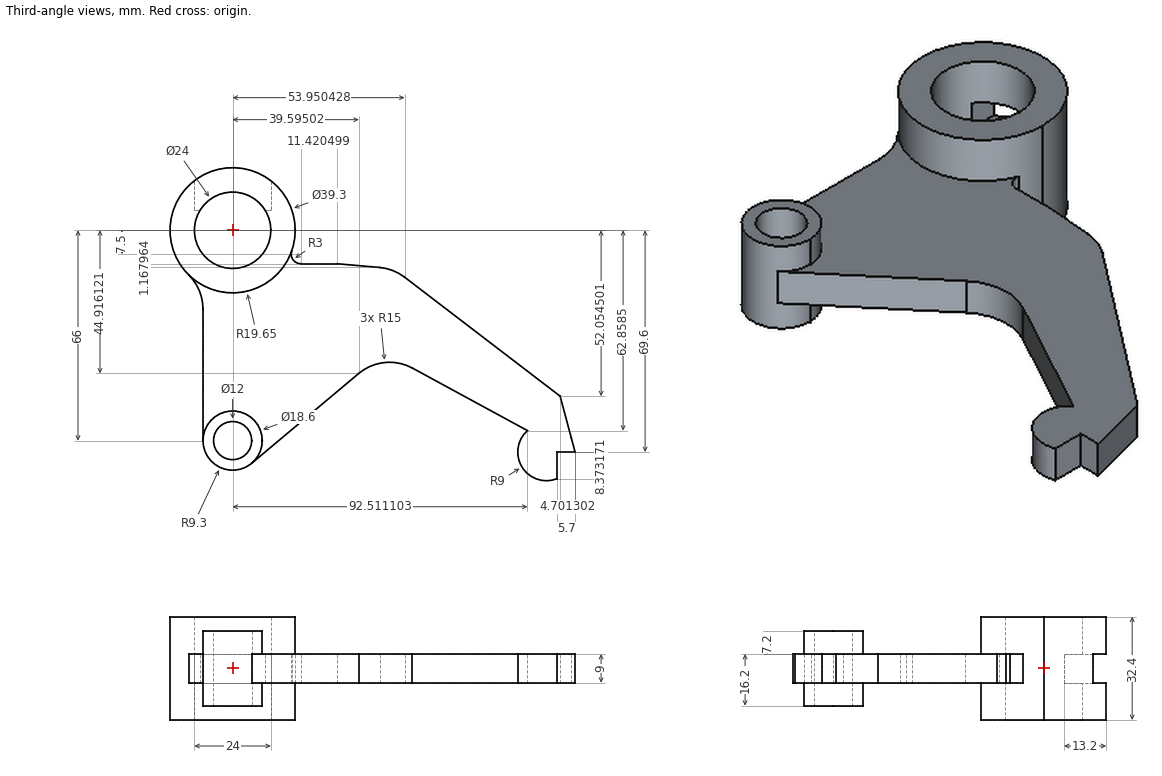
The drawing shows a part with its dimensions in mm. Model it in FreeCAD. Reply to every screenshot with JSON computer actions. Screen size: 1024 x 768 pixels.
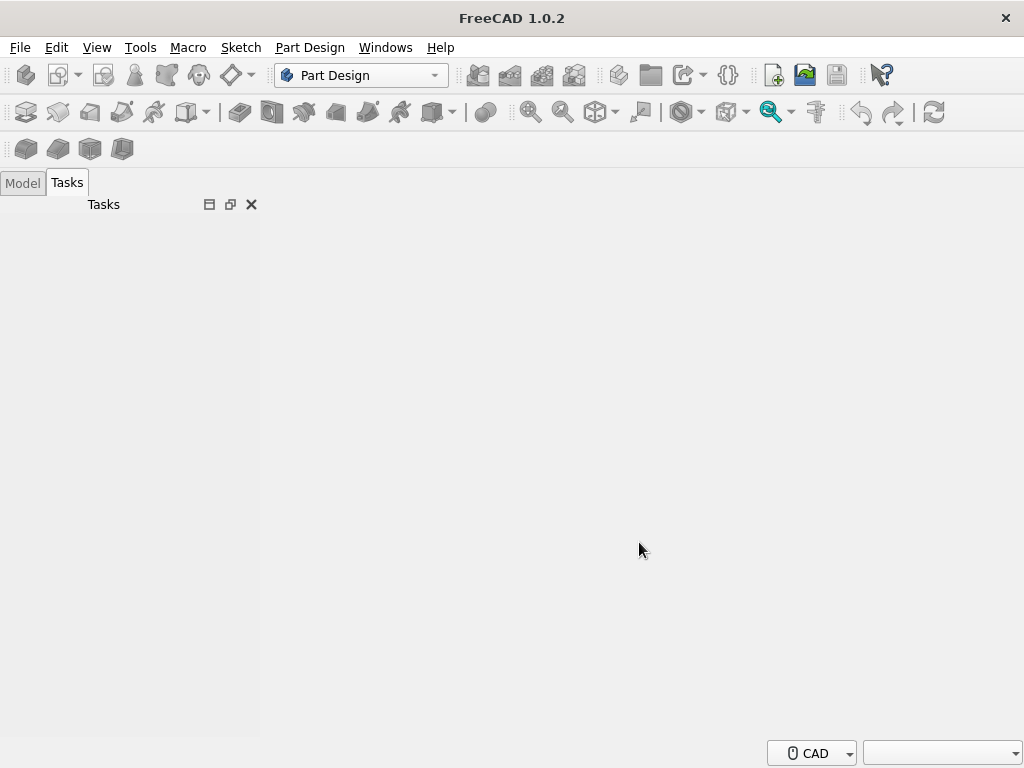
{"action": "key", "text": "ctrl+n"}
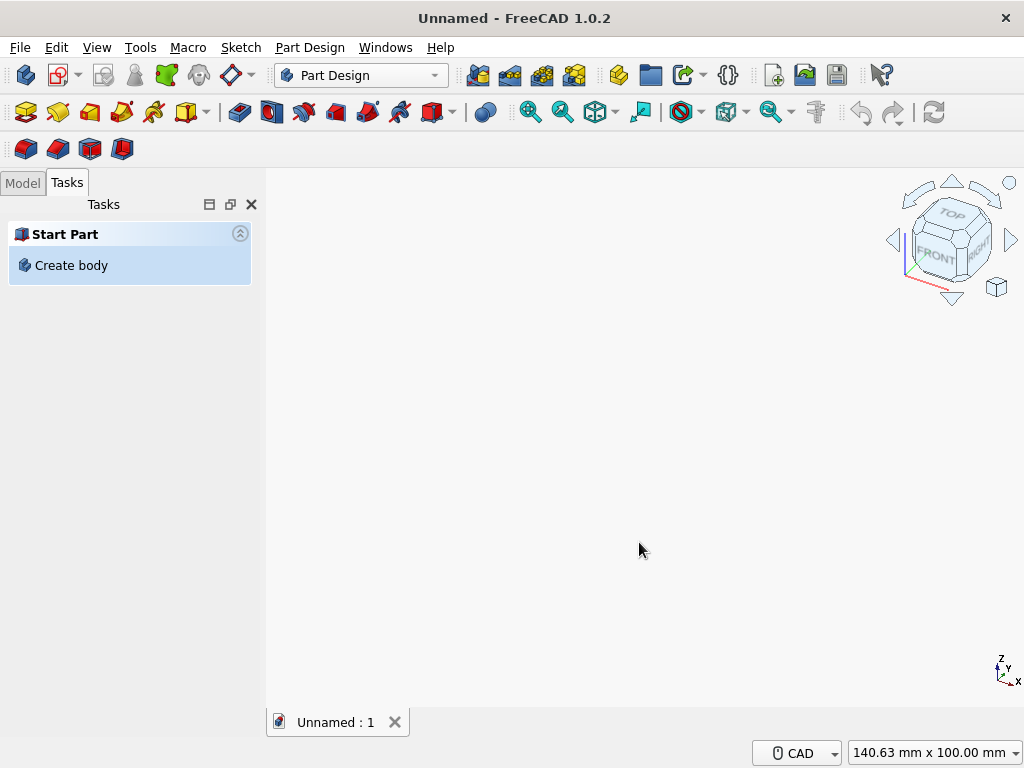
{"action": "left_click", "coordinate": [58, 76]}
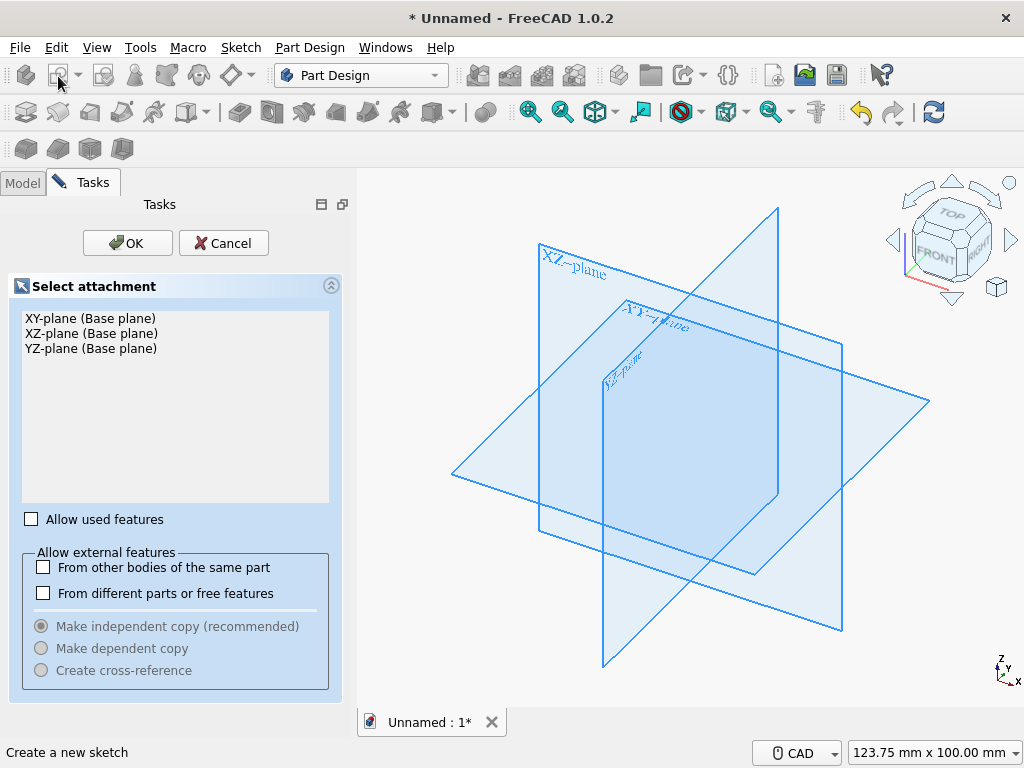
{"action": "left_click", "coordinate": [82, 318]}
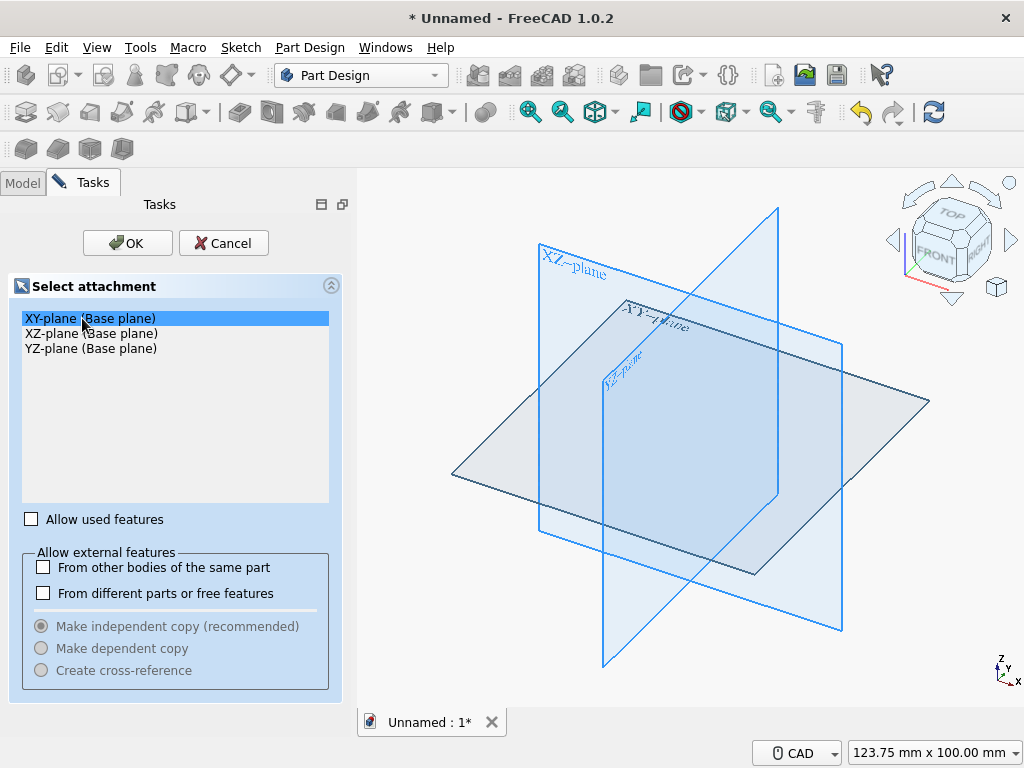
{"action": "left_click", "coordinate": [128, 243]}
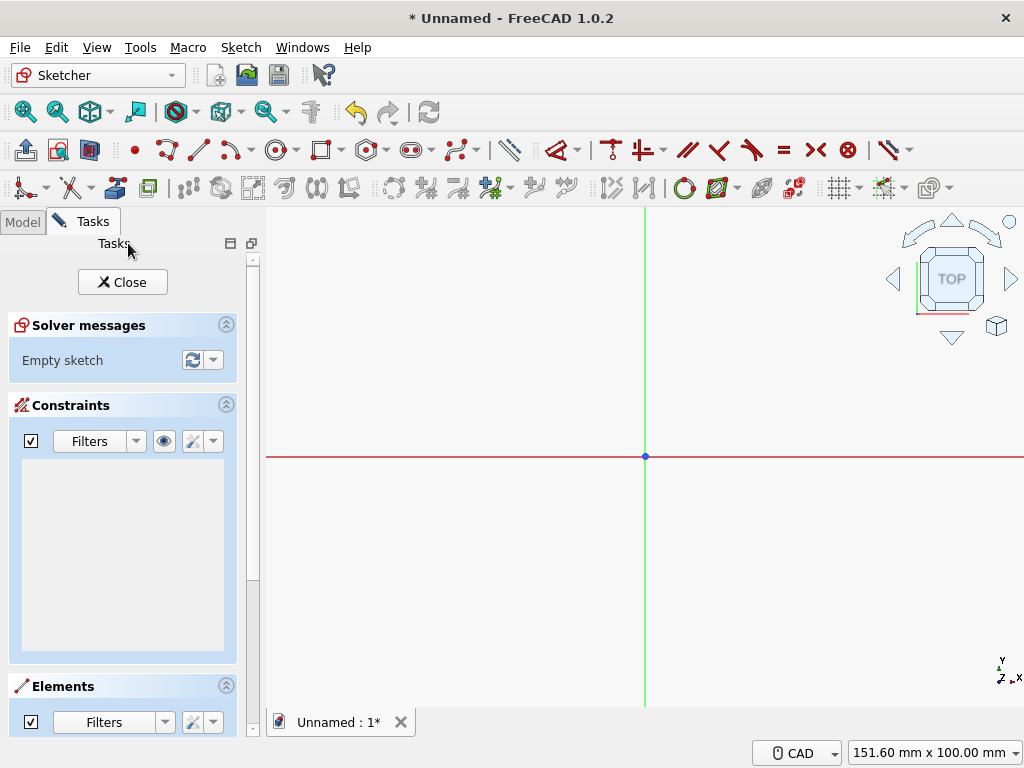
{"action": "scroll", "coordinate": [784, 457], "scroll_direction": "up", "scroll_amount": 2}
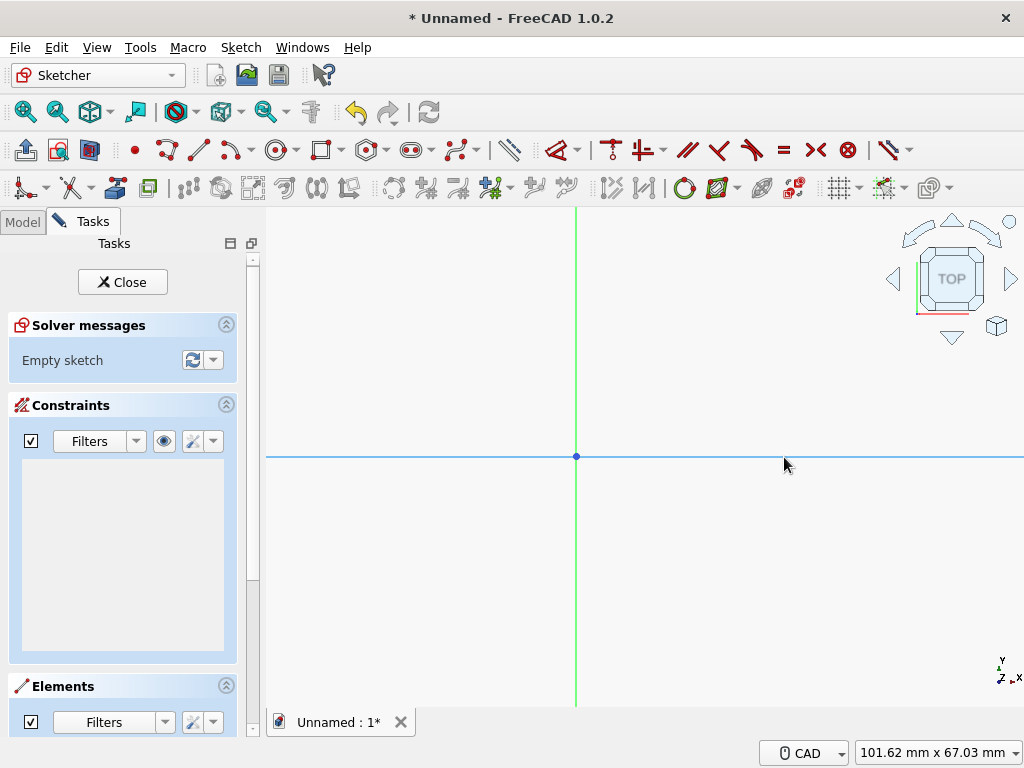
{"action": "left_click", "coordinate": [276, 150]}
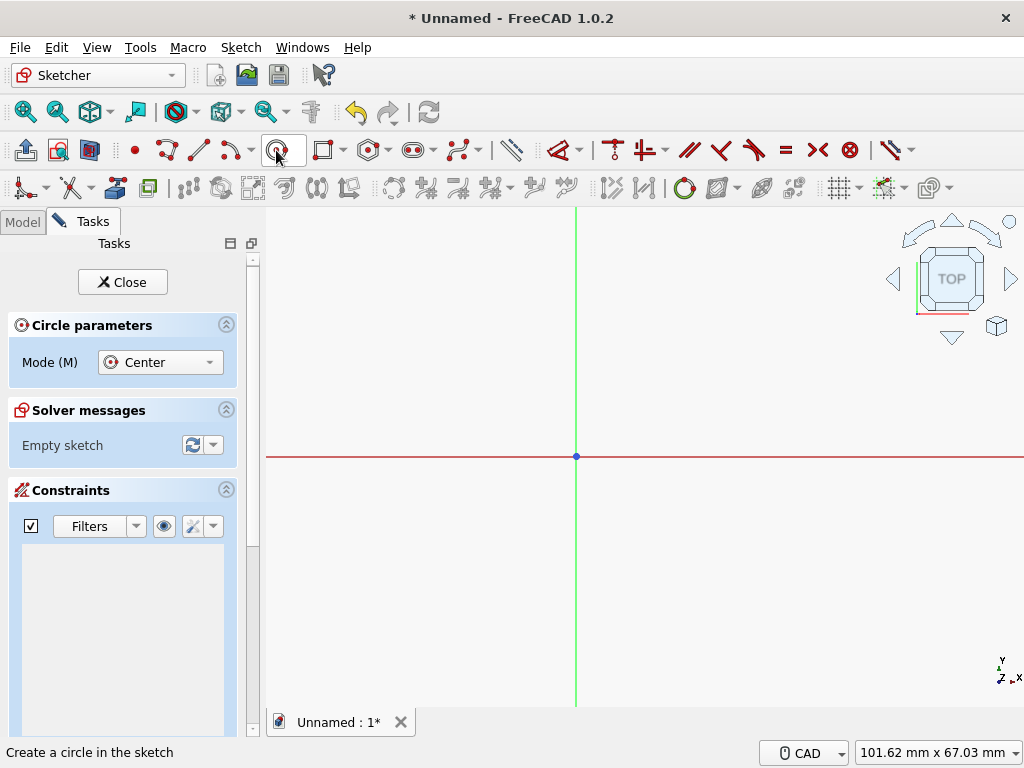
{"action": "left_click", "coordinate": [576, 457]}
{"action": "mouse_move", "coordinate": [680, 353]}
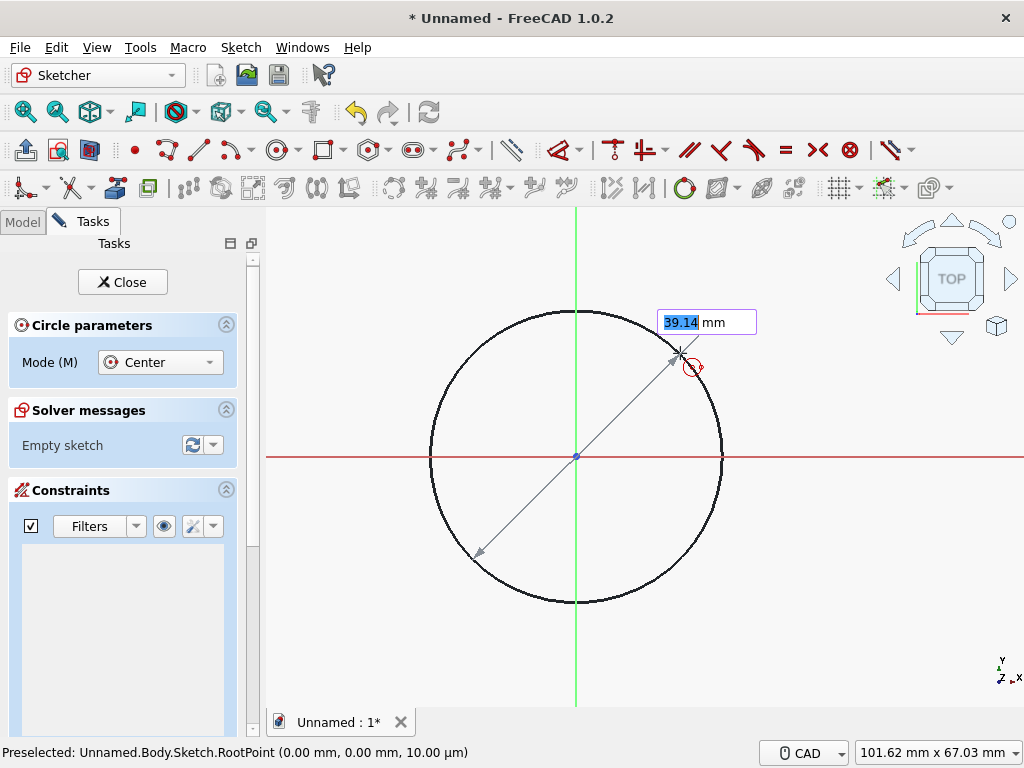
{"action": "type", "text": "39.3"}
{"action": "key", "text": "Return"}
{"action": "key", "text": "Escape"}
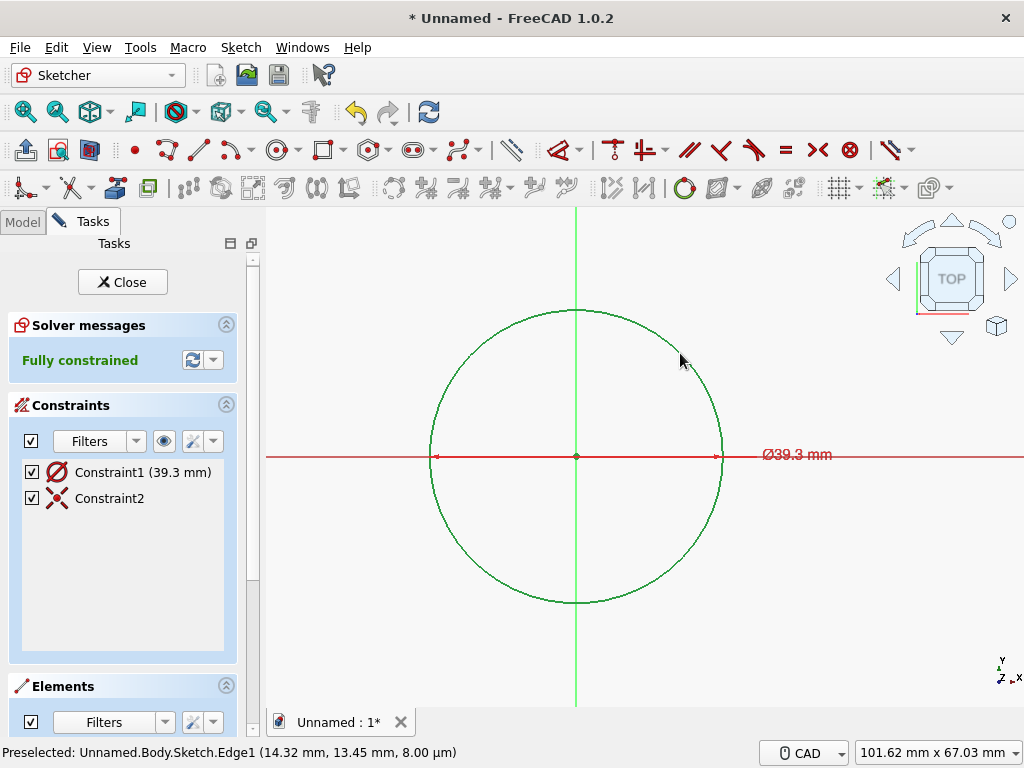
{"action": "left_click", "coordinate": [123, 282]}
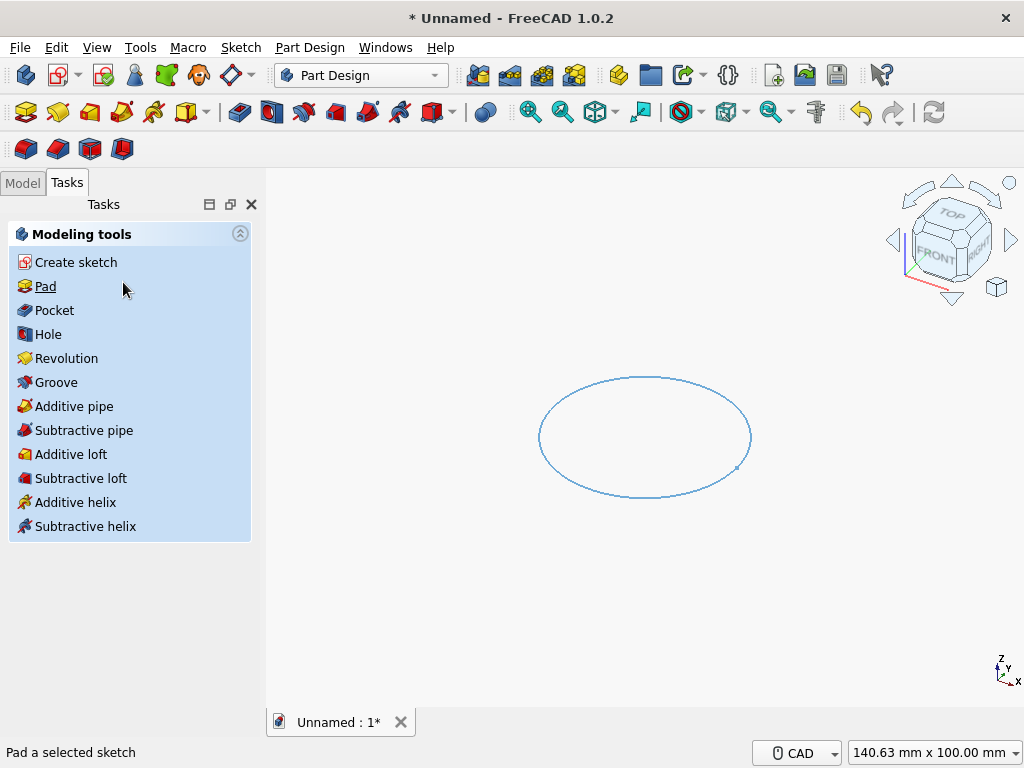
{"action": "left_click", "coordinate": [26, 112]}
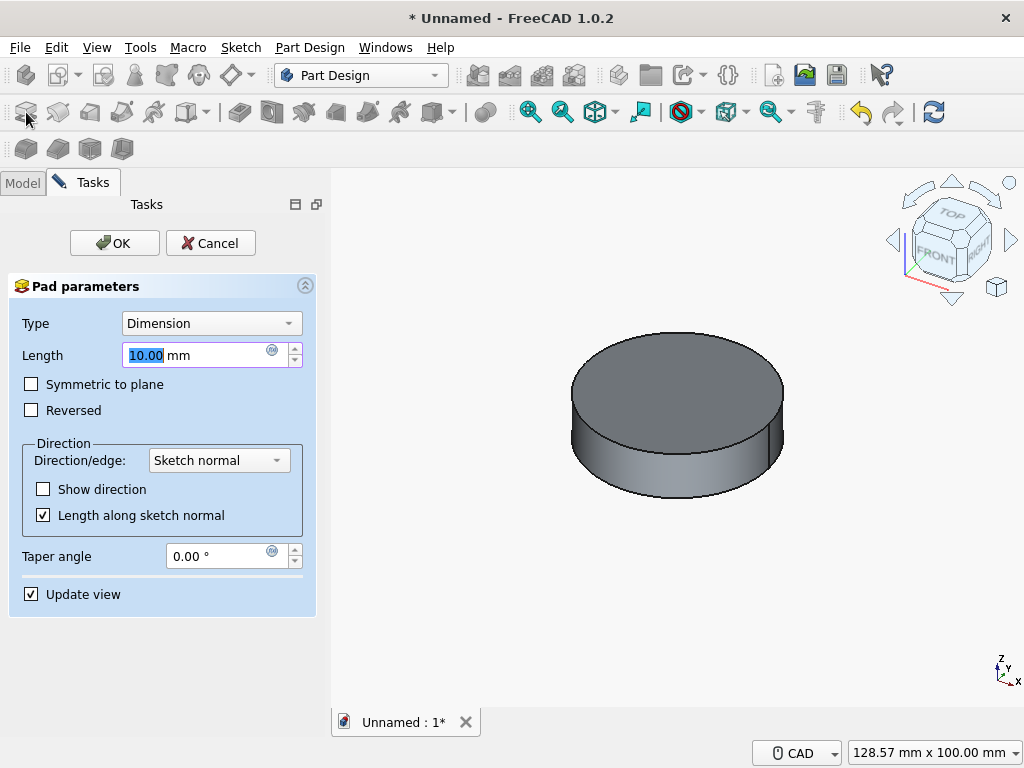
{"action": "type", "text": "32.4"}
{"action": "key", "text": "Tab"}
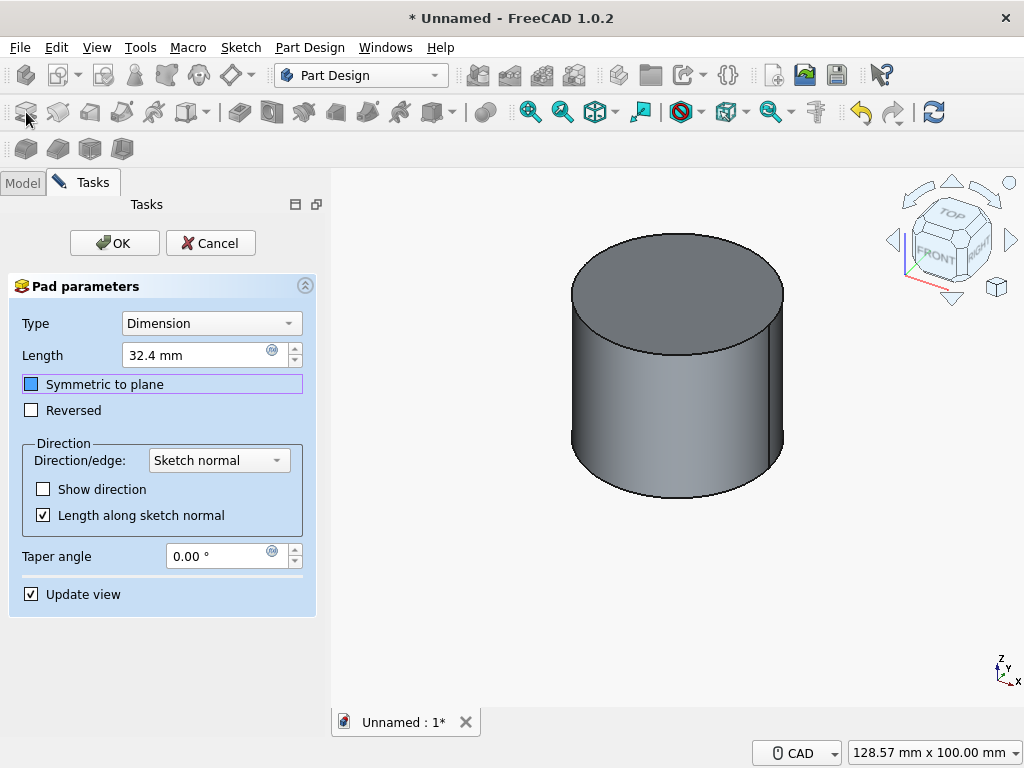
{"action": "left_click", "coordinate": [30, 384]}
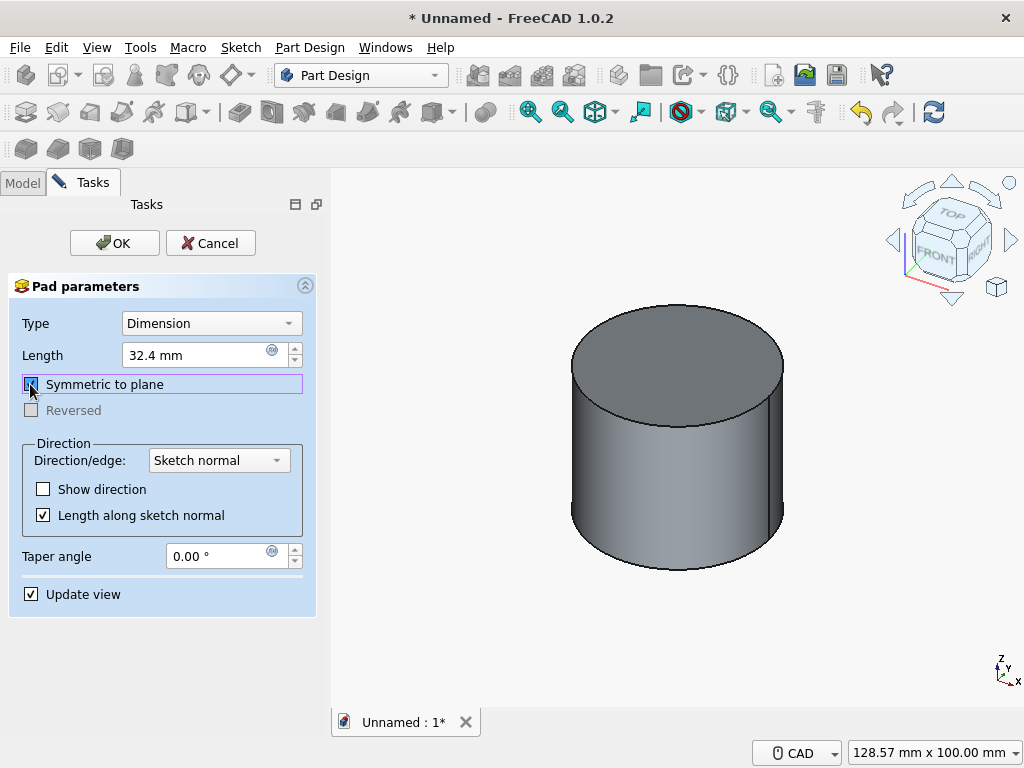
{"action": "left_click", "coordinate": [115, 243]}